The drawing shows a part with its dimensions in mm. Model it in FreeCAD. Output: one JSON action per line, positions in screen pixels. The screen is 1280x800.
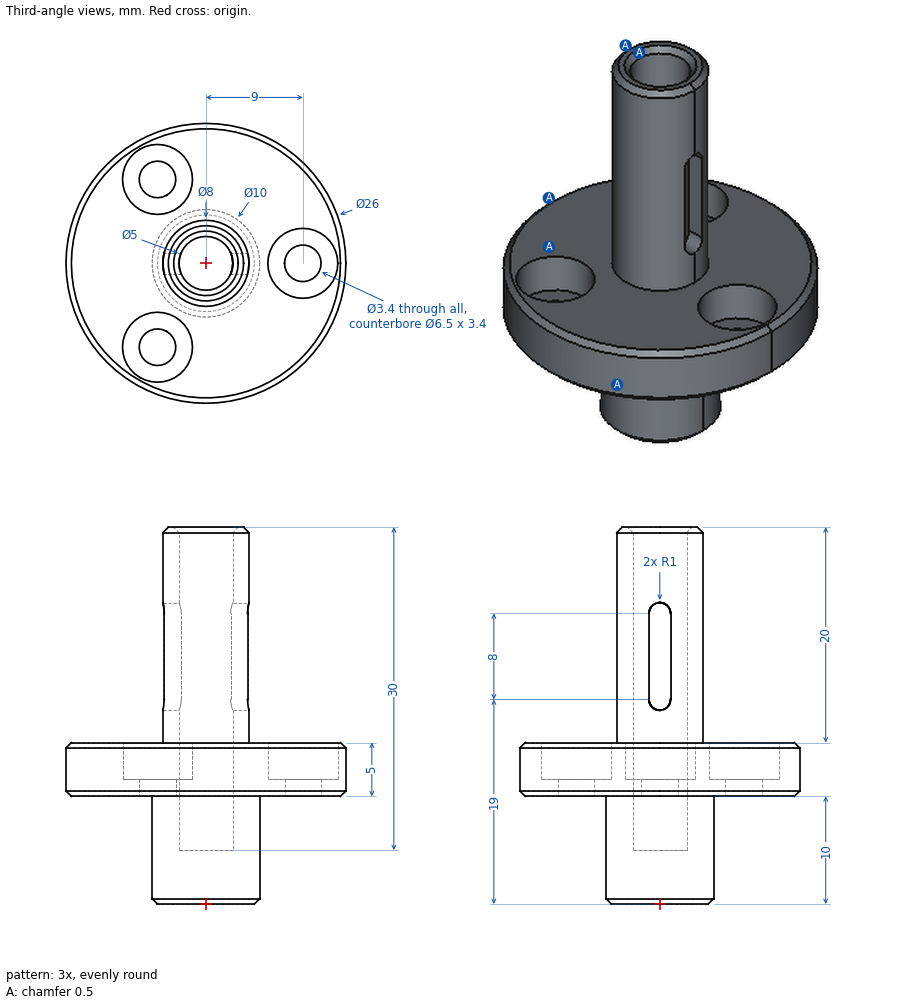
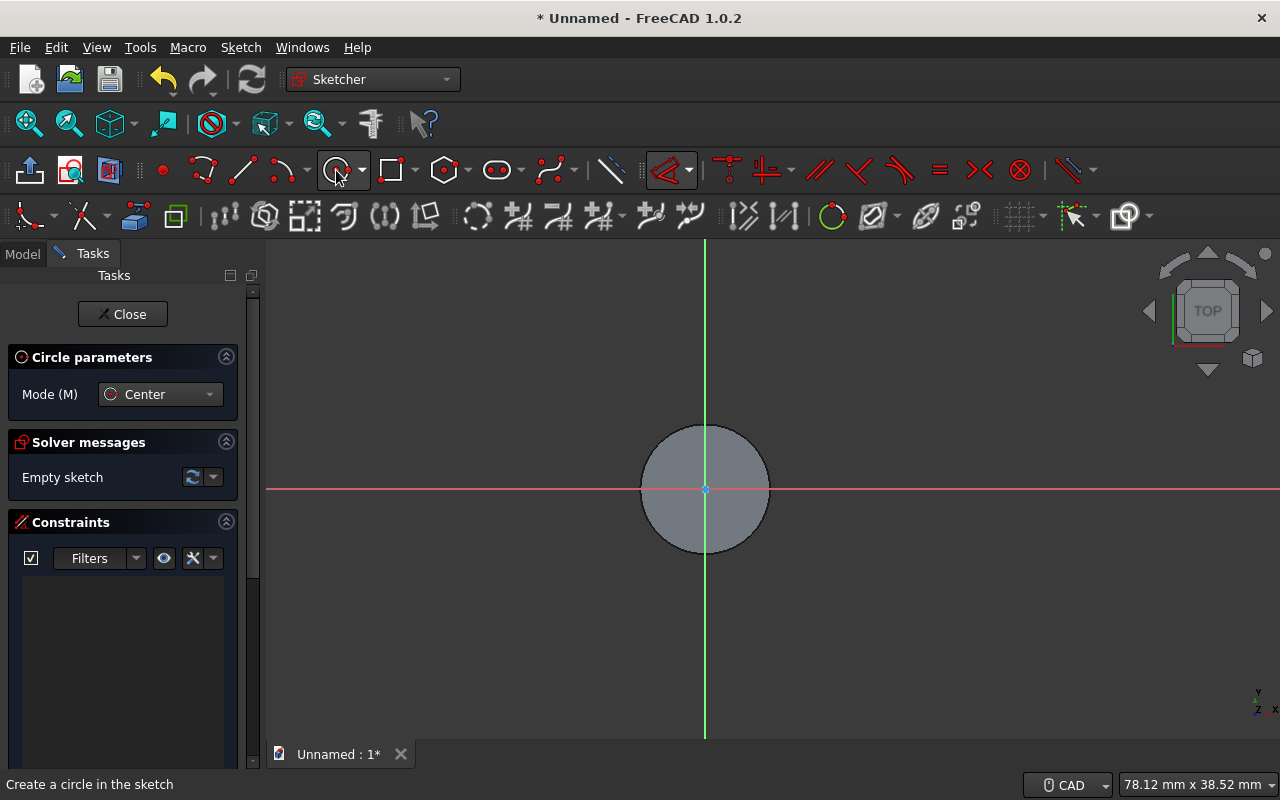
{"action": "left_click", "coordinate": [705, 489]}
{"action": "left_click", "coordinate": [825, 370]}
{"action": "key", "text": "Escape"}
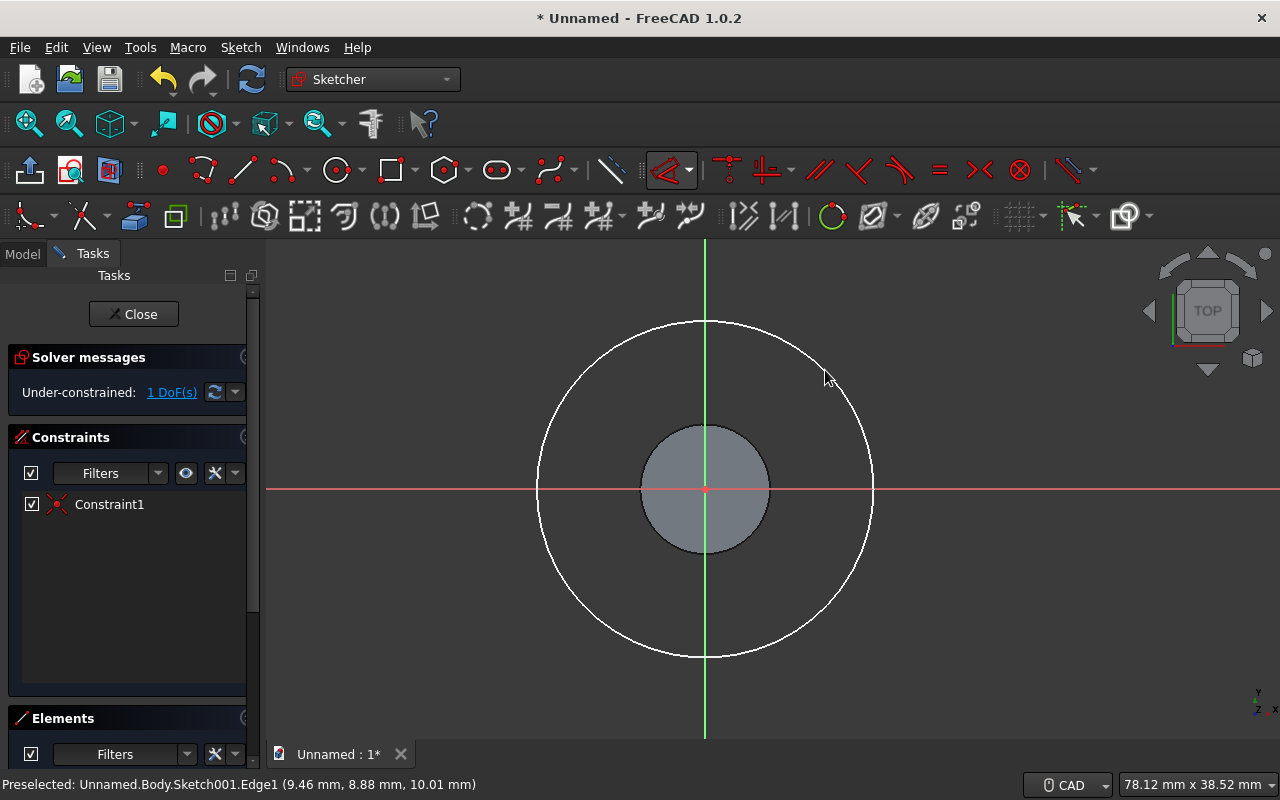
{"action": "left_click", "coordinate": [824, 370]}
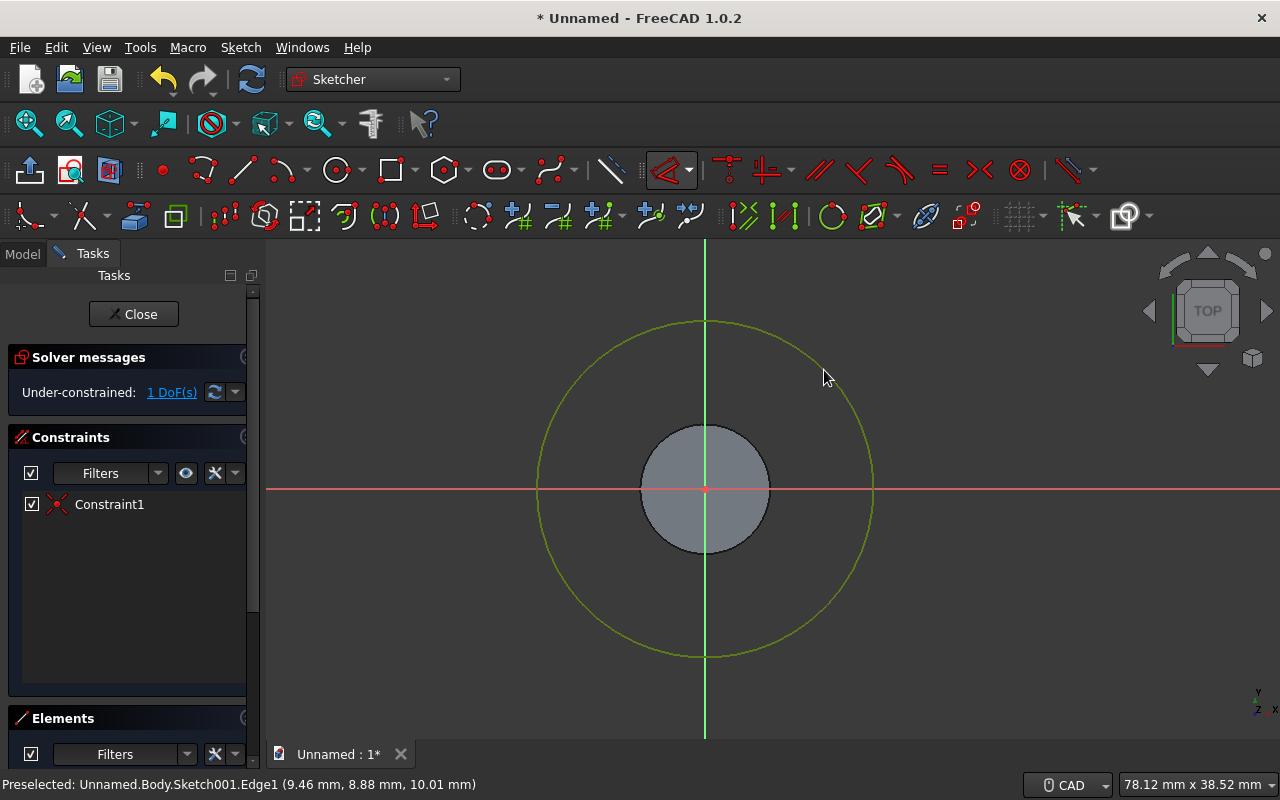
{"action": "key", "text": "k o"}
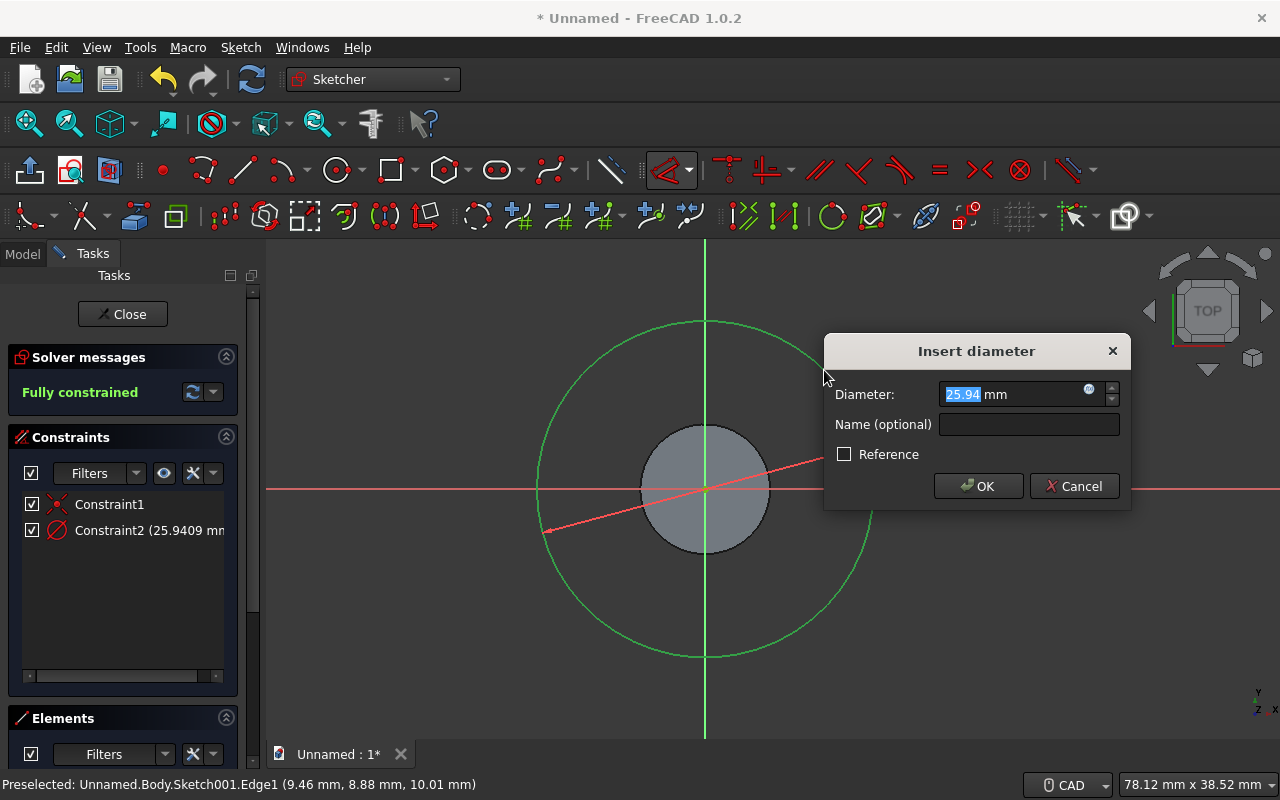
{"action": "type", "text": "26"}
{"action": "key", "text": "Return"}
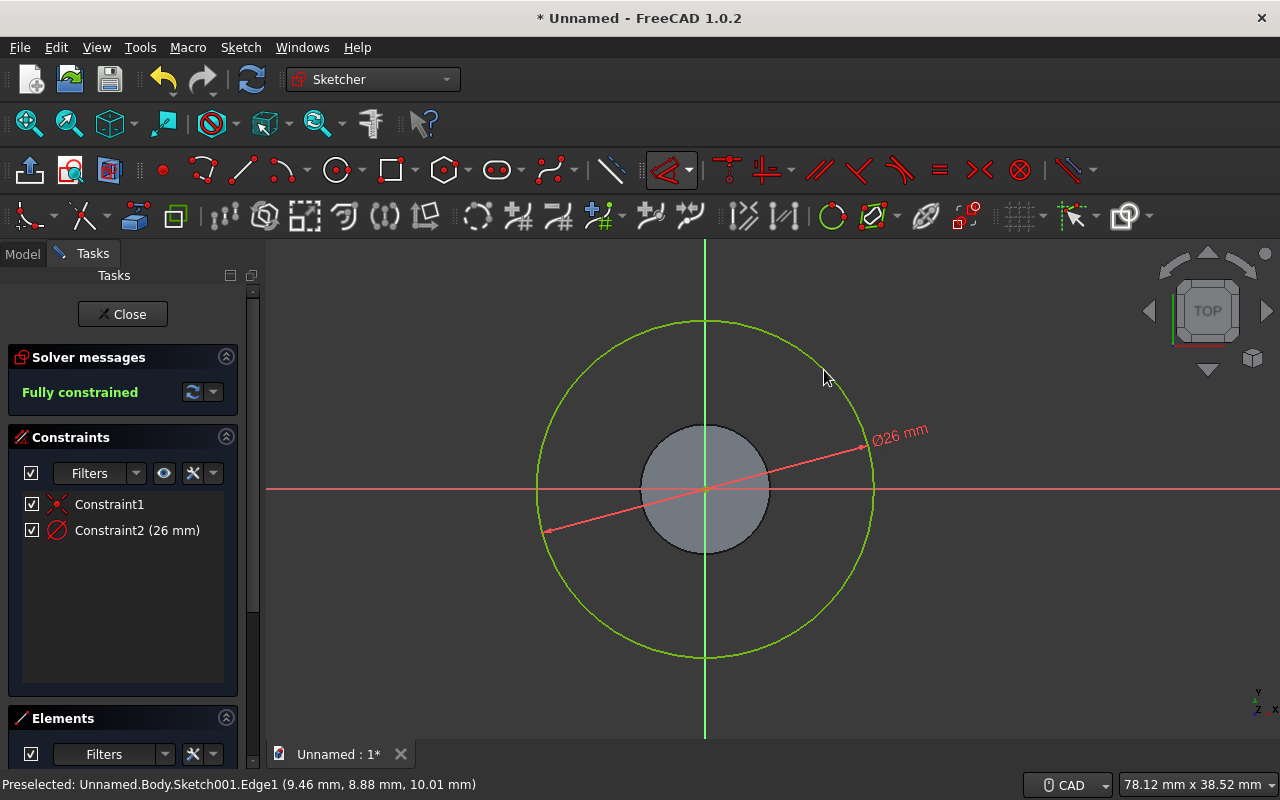
{"action": "left_click", "coordinate": [123, 314]}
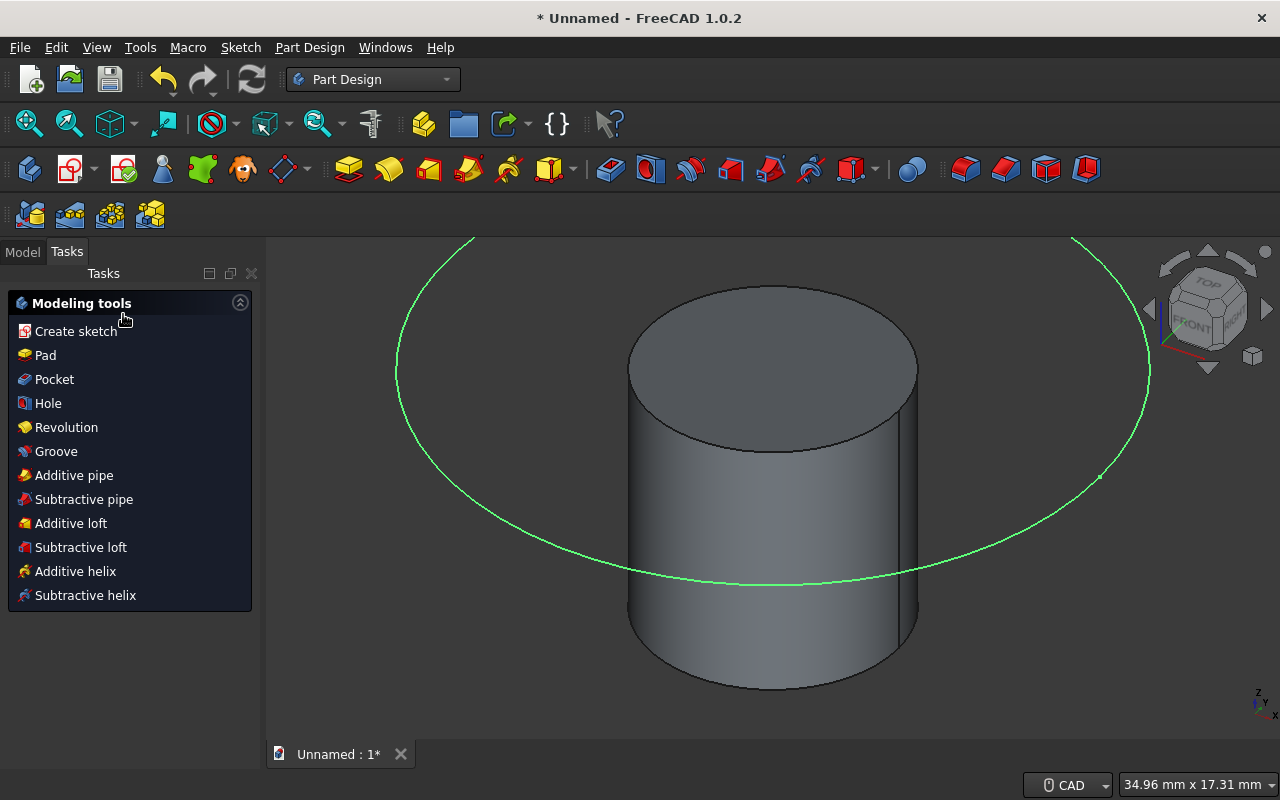
{"action": "left_click", "coordinate": [350, 170]}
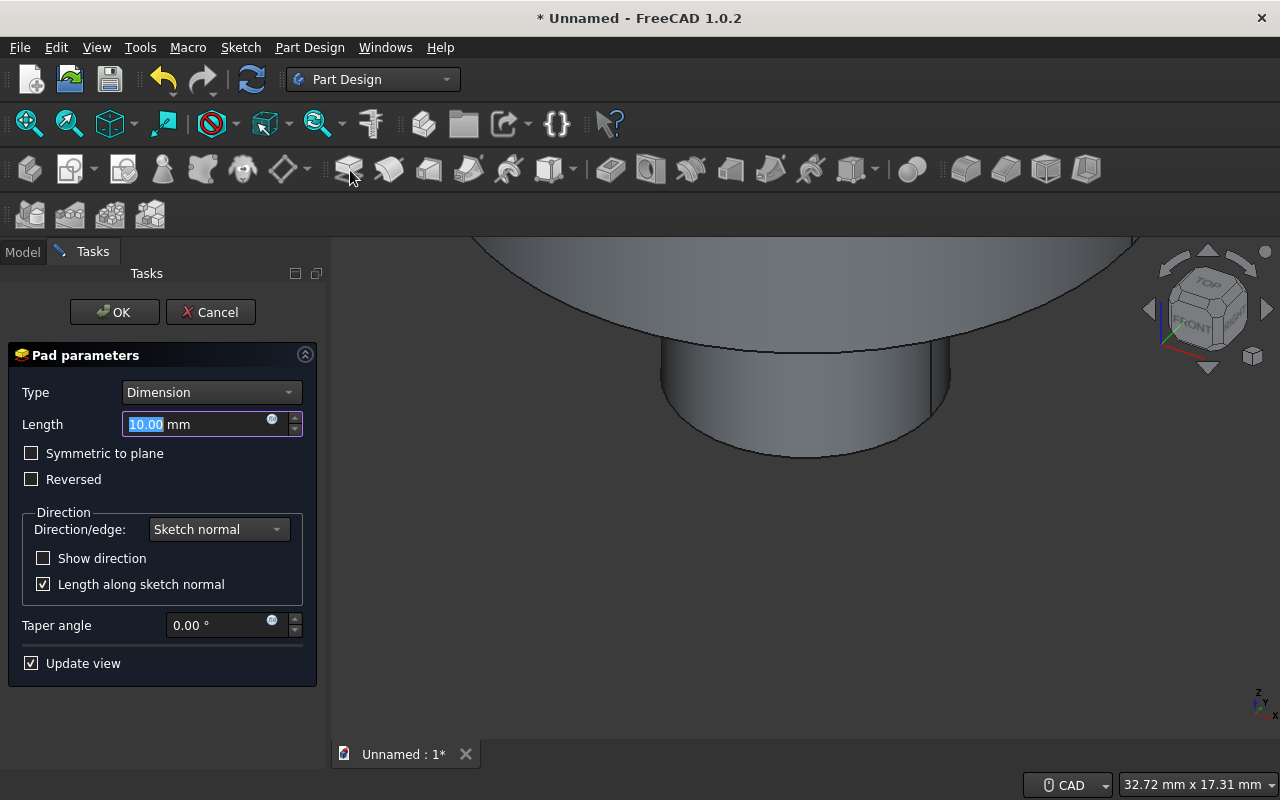
{"action": "type", "text": "5"}
{"action": "key", "text": "Tab"}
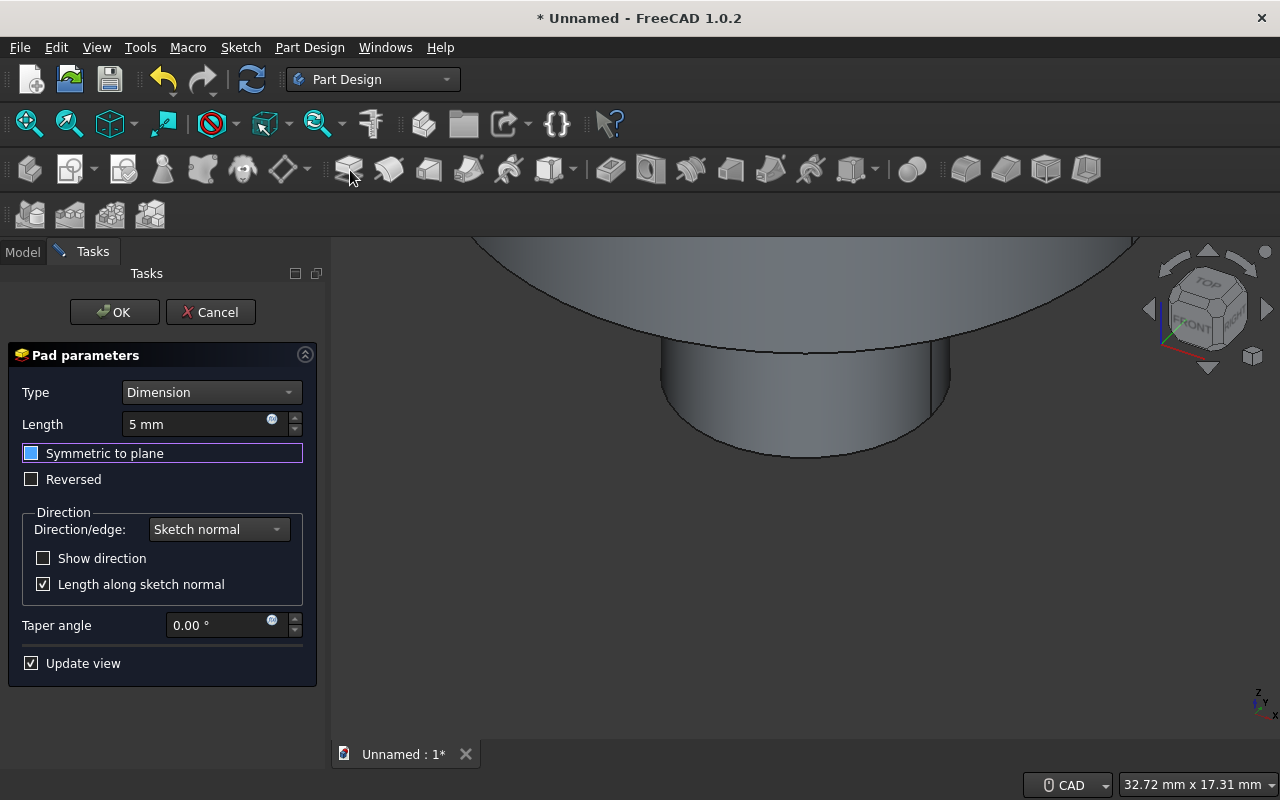
{"action": "left_click", "coordinate": [115, 312]}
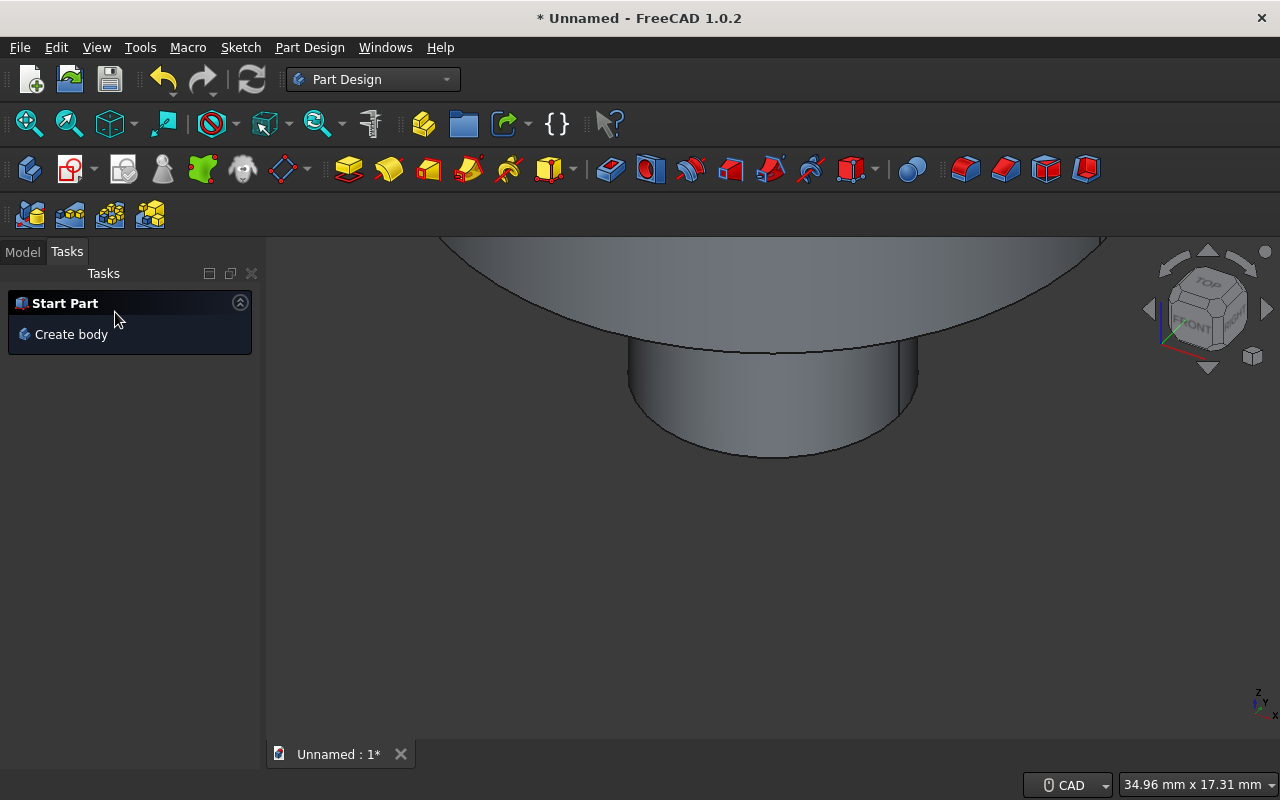
{"action": "left_click", "coordinate": [30, 124]}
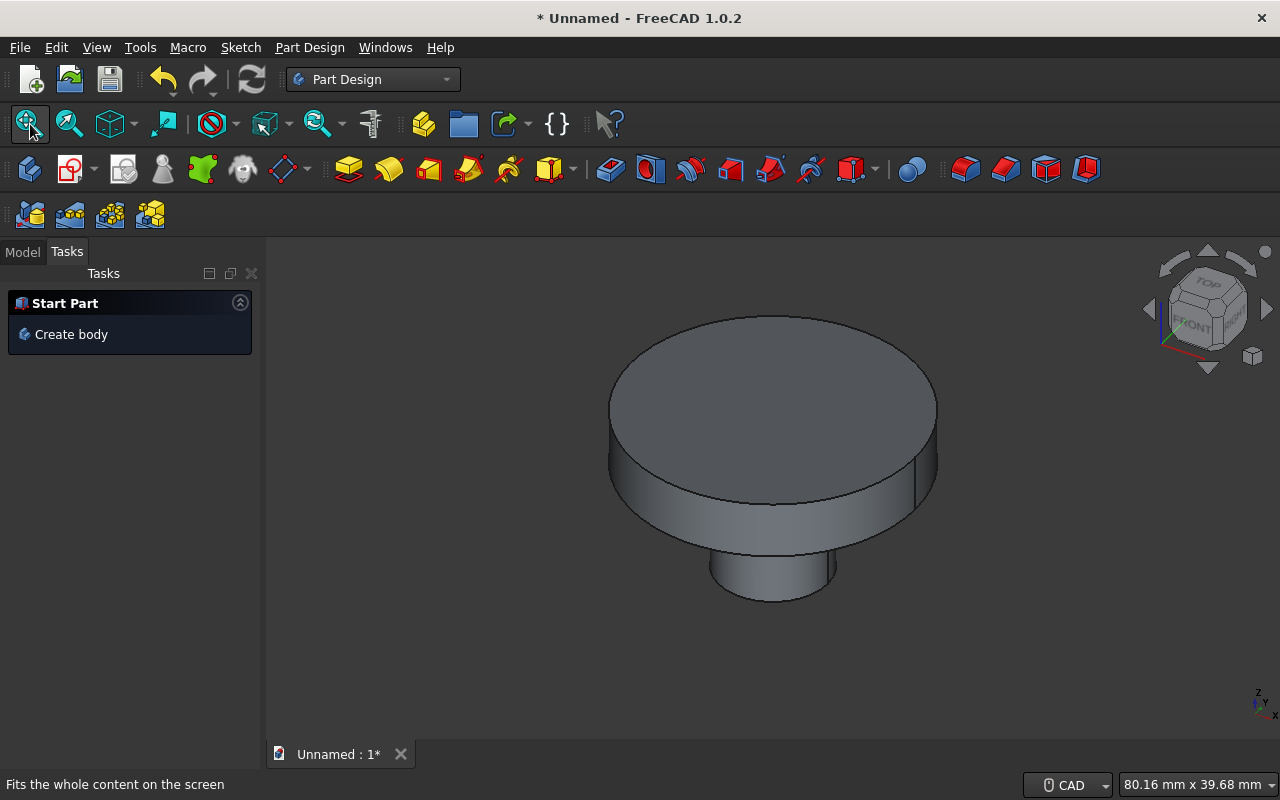
{"action": "left_click", "coordinate": [773, 409]}